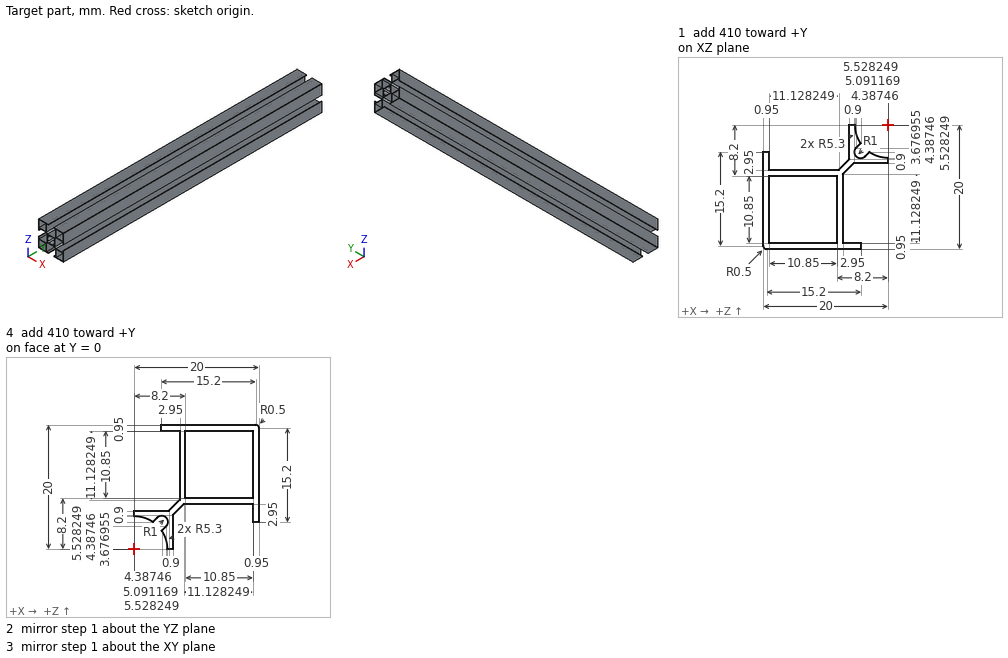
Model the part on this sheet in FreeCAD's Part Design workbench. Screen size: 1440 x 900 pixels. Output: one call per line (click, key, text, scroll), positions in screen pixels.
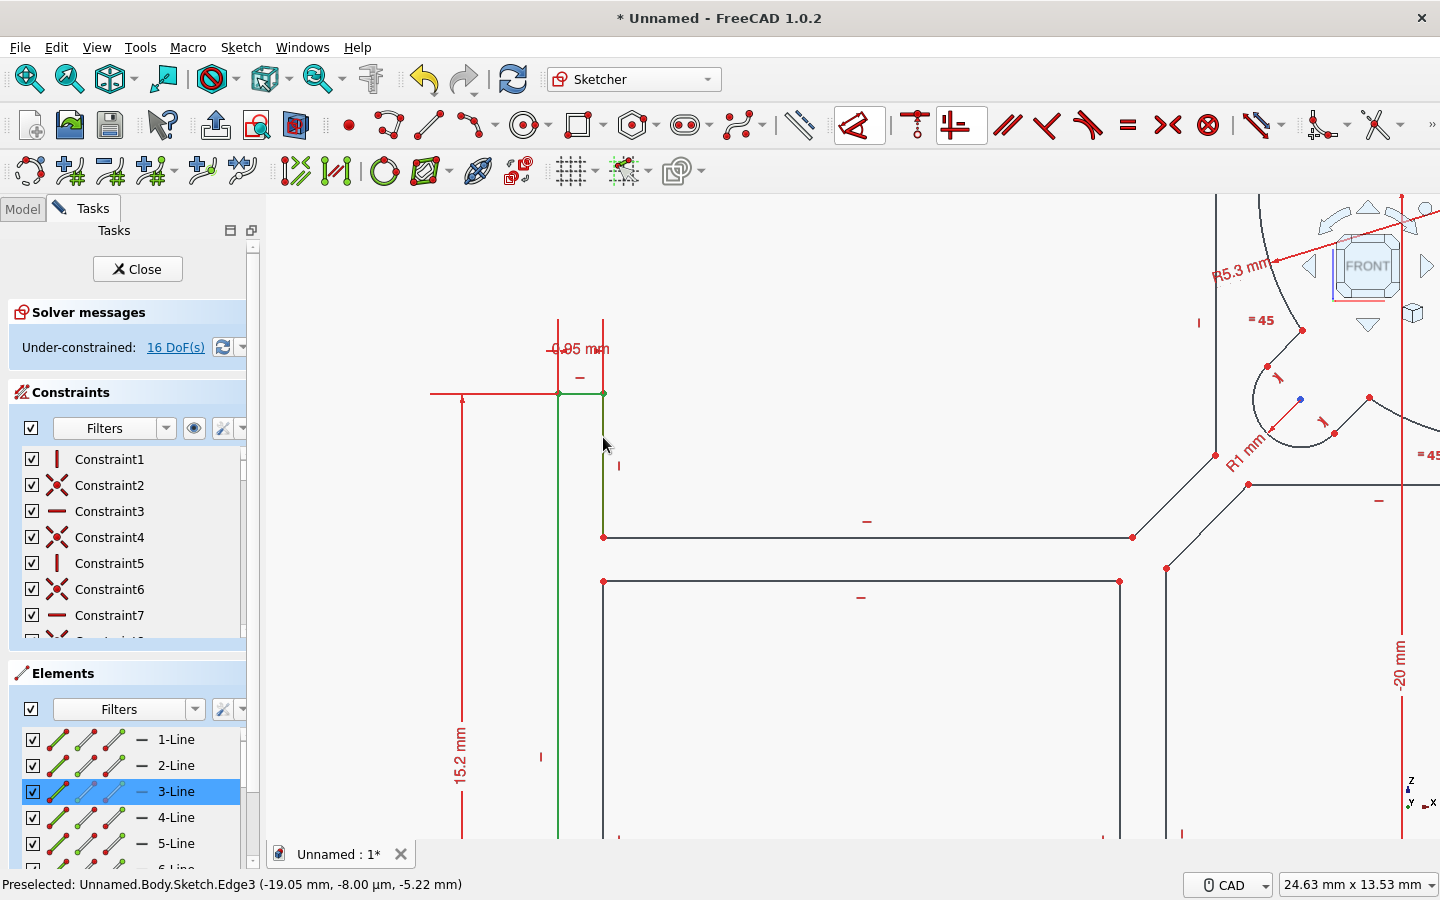
key(i)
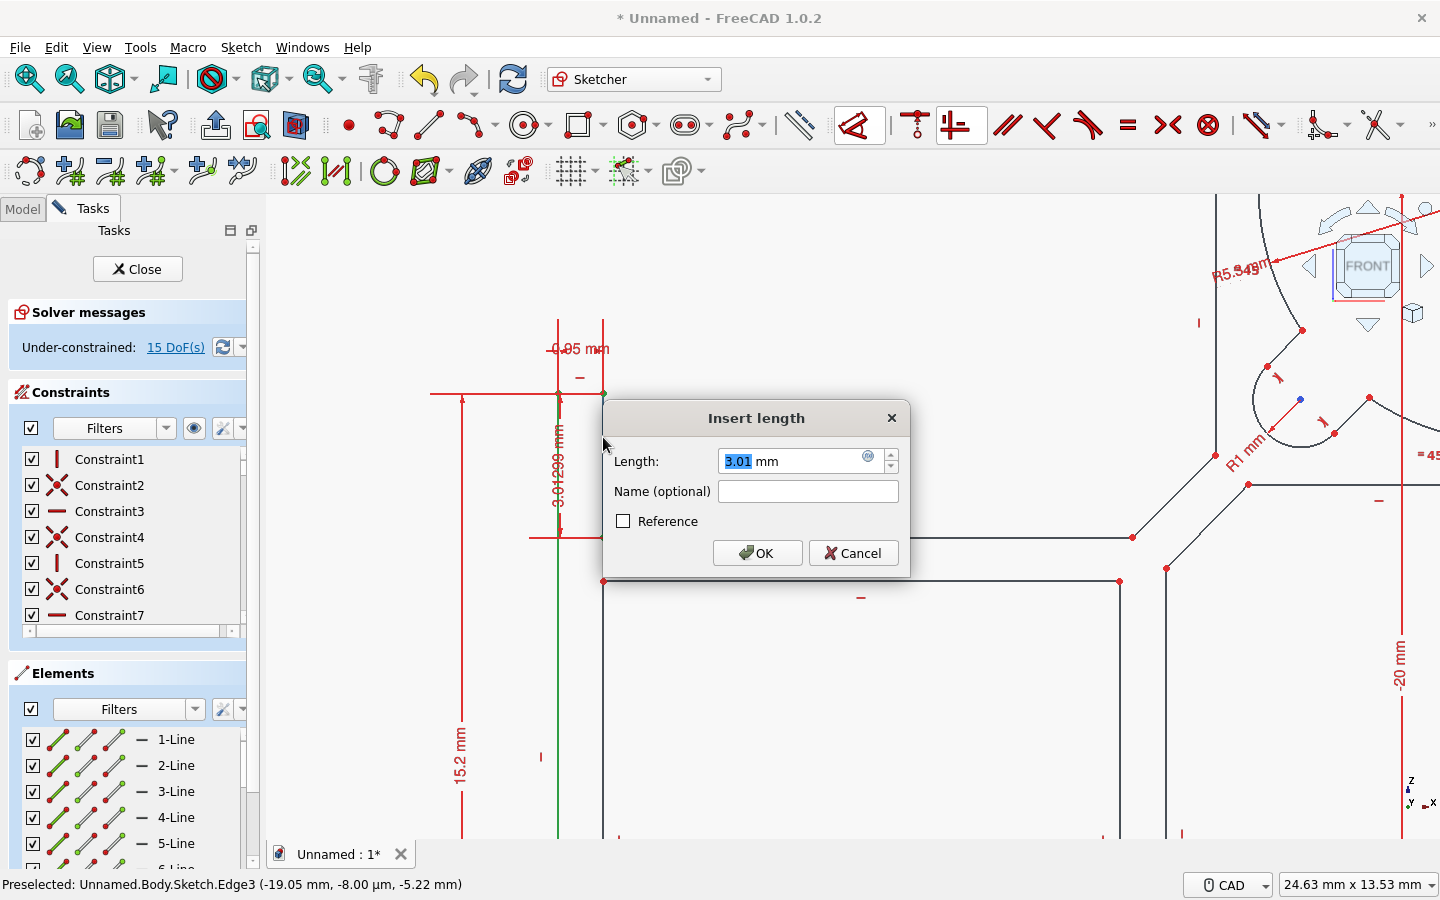
text(2.95)
key(Return)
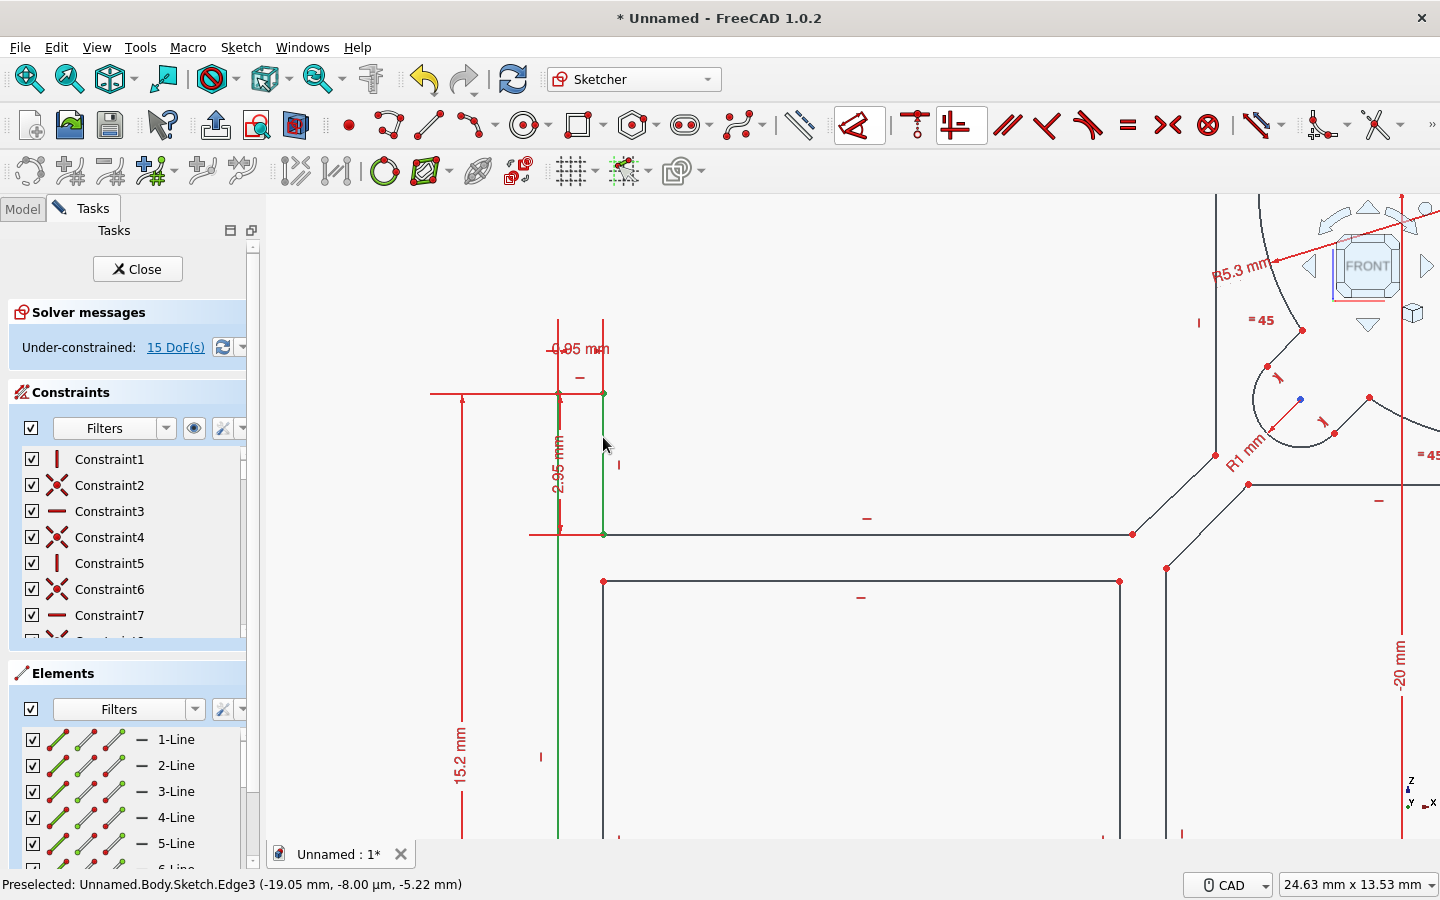
scroll(580, 395, down, 4)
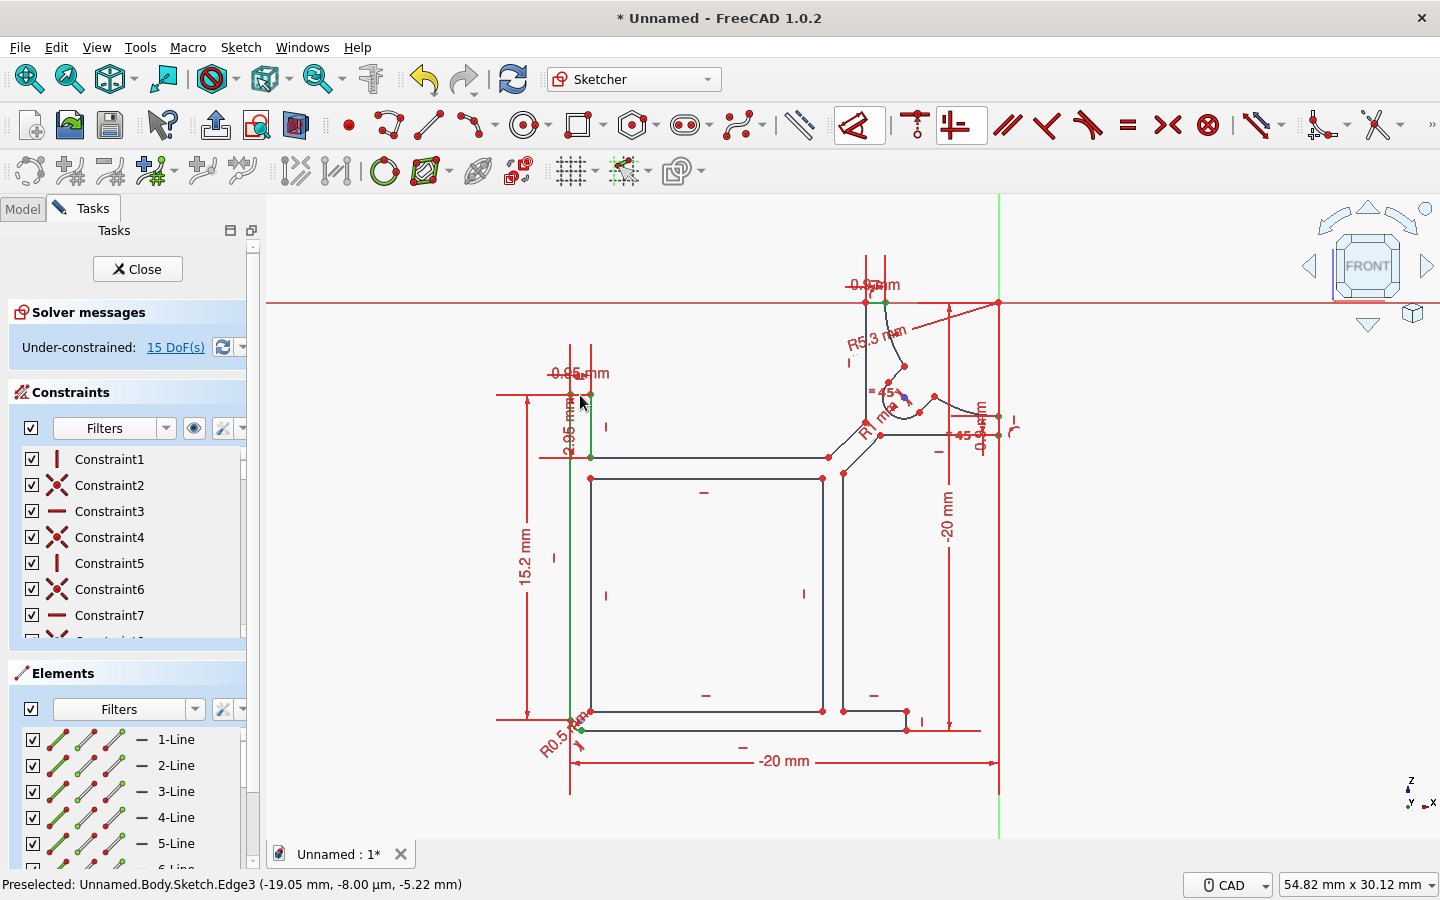
click(888, 711)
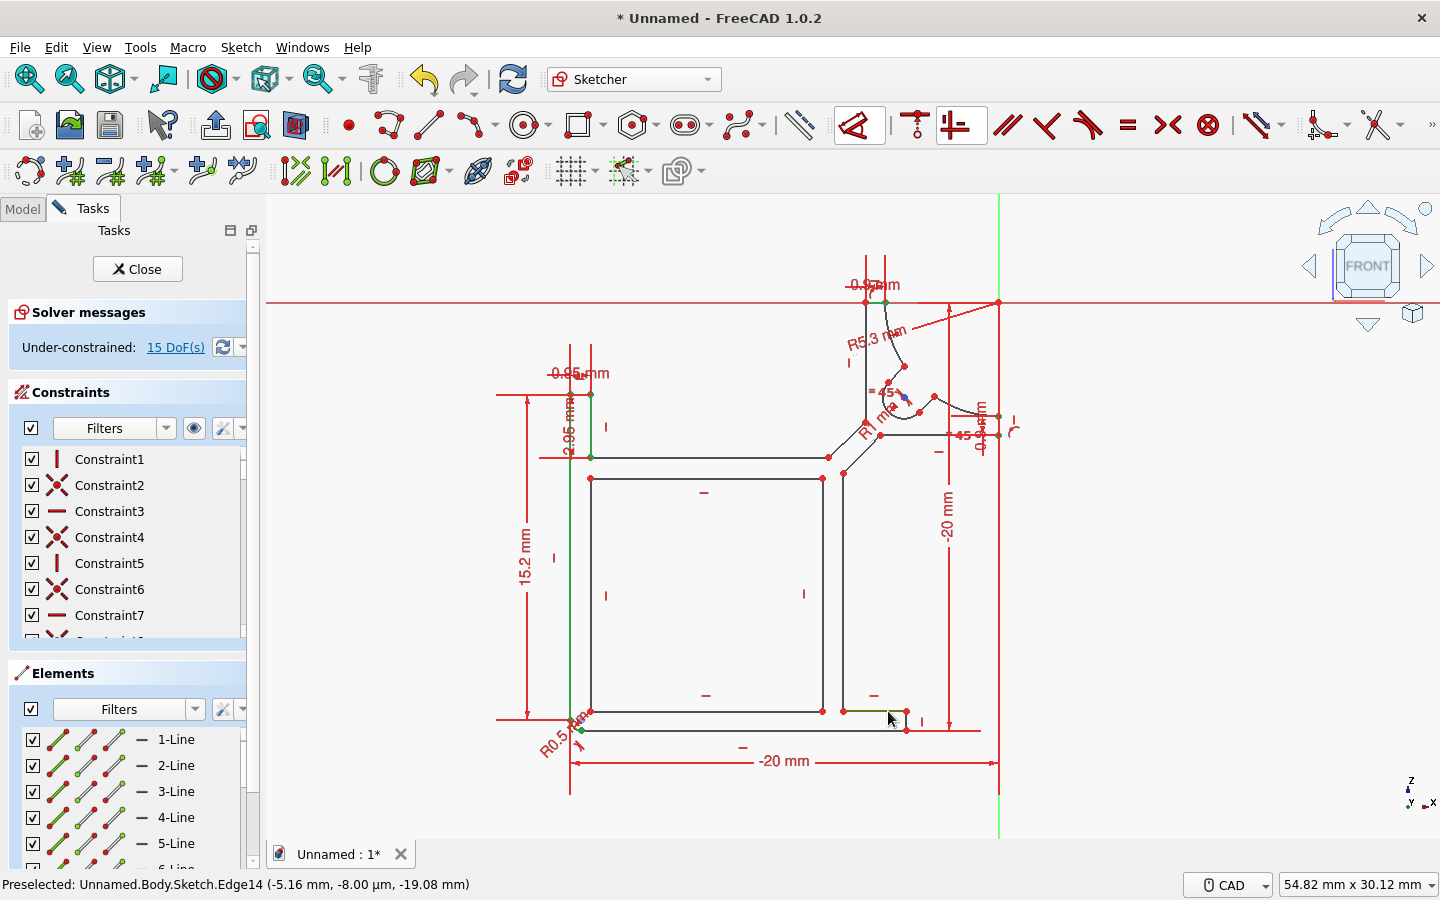
click(880, 126)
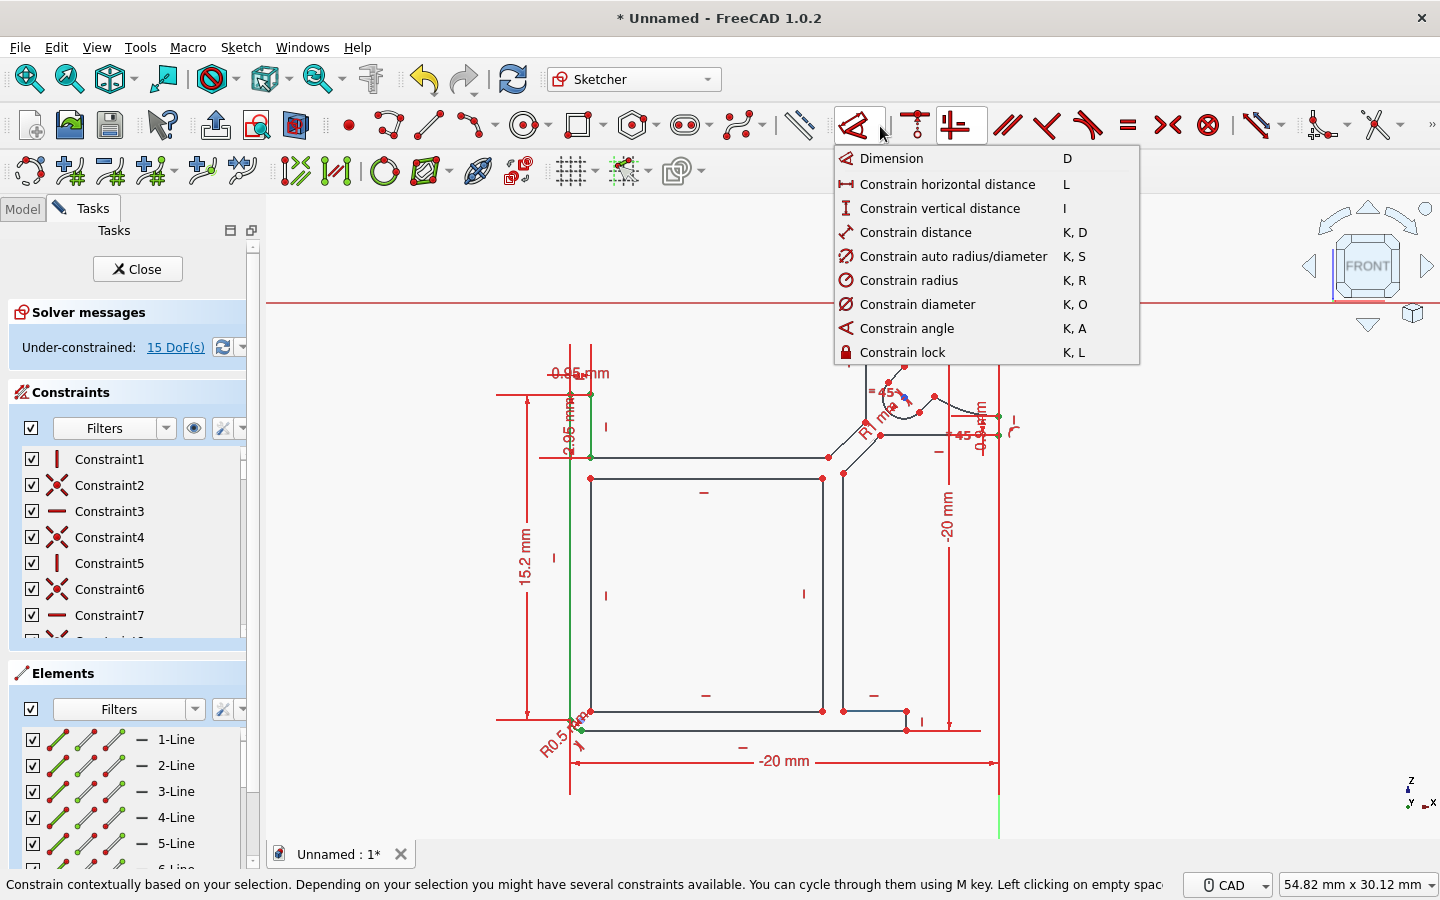
click(987, 184)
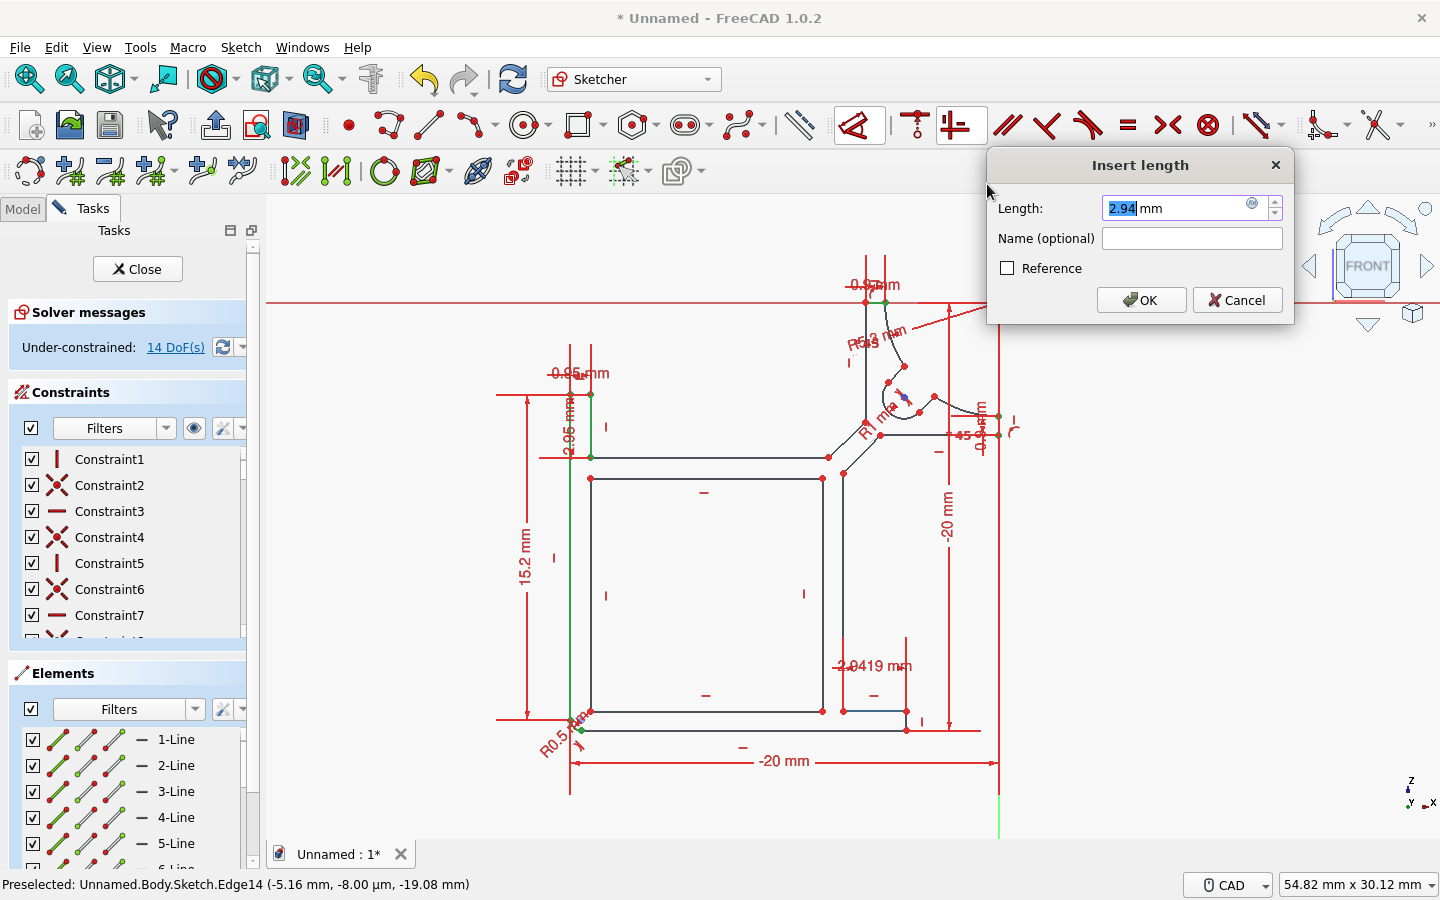
text(2.95)
key(Return)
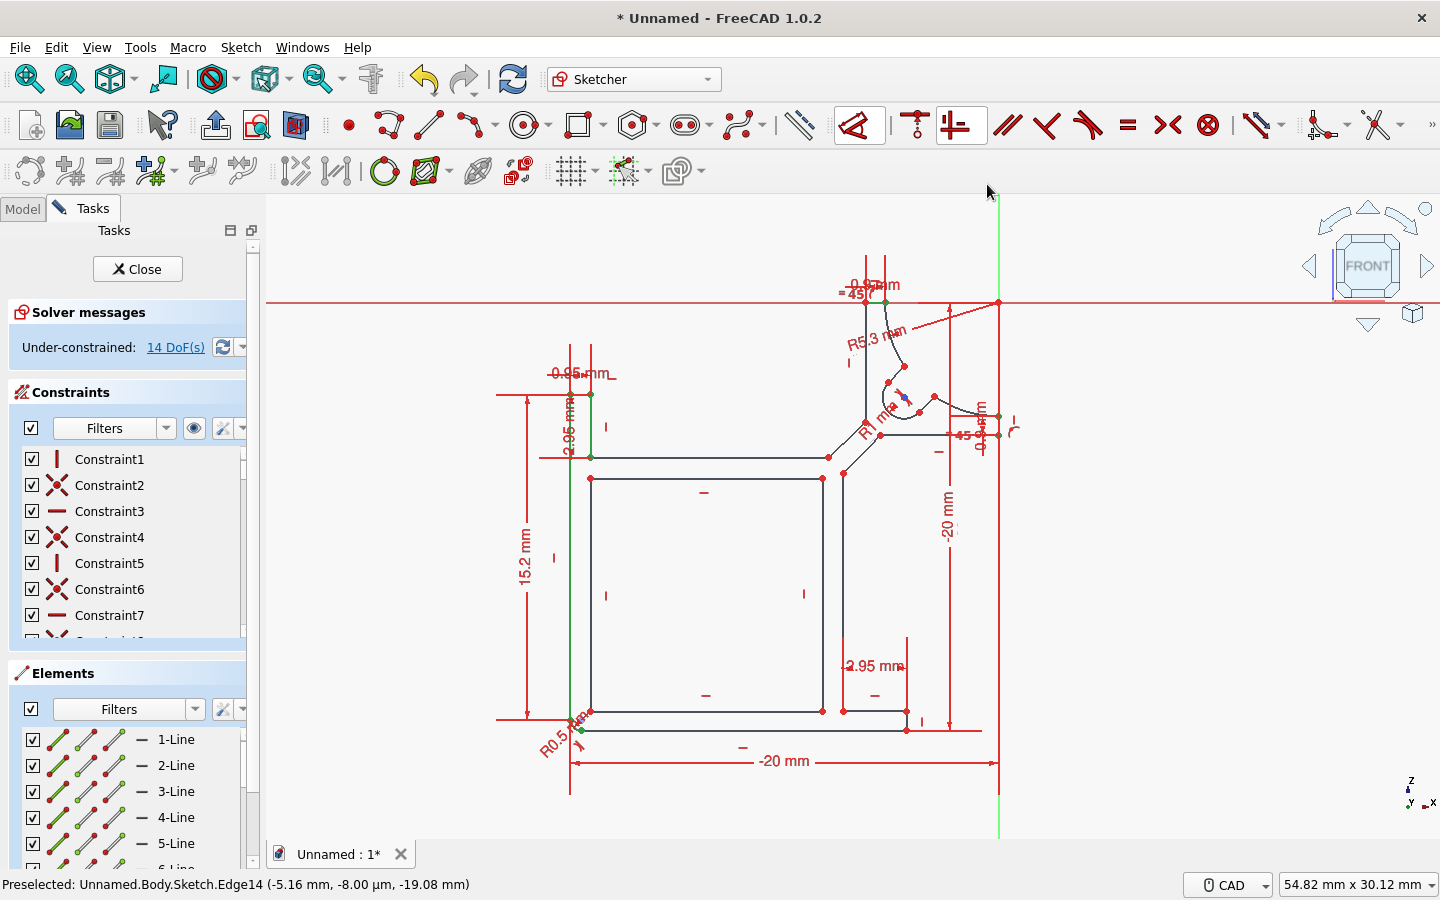
scroll(907, 721, up, 4)